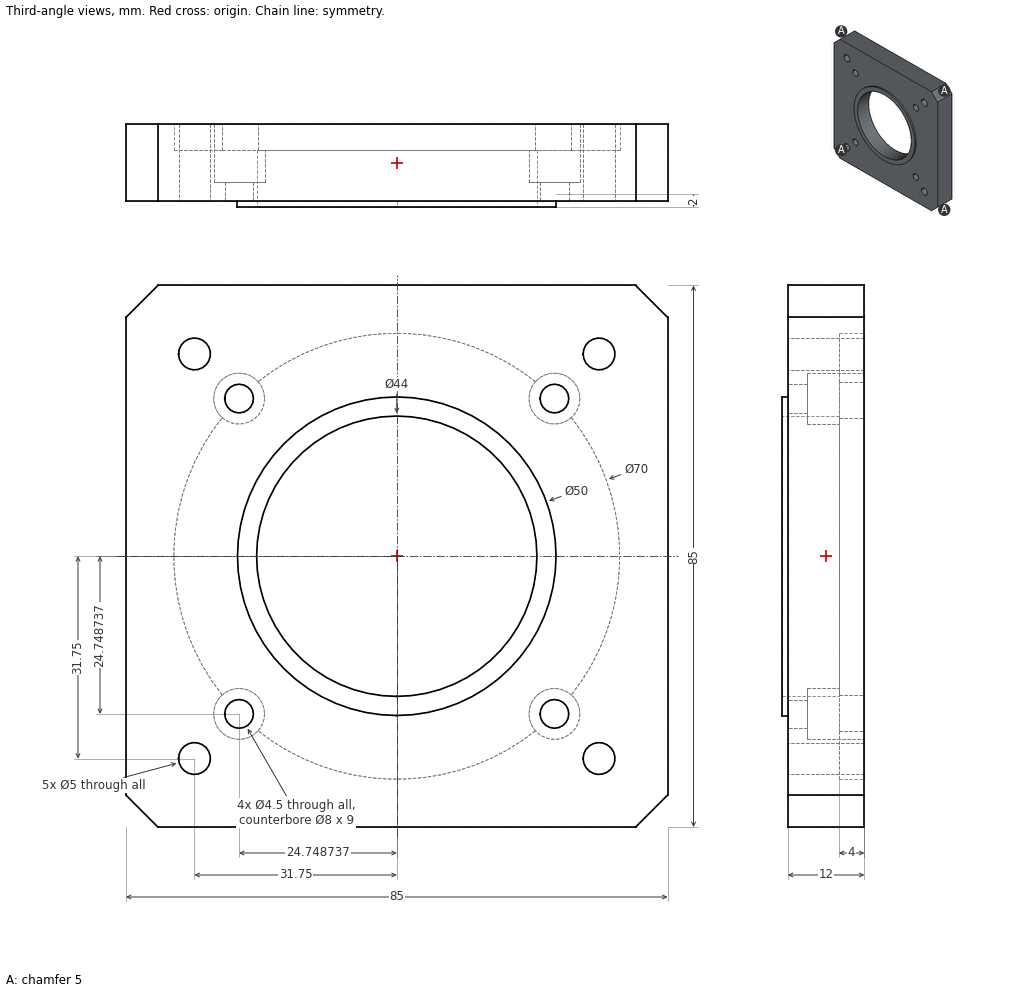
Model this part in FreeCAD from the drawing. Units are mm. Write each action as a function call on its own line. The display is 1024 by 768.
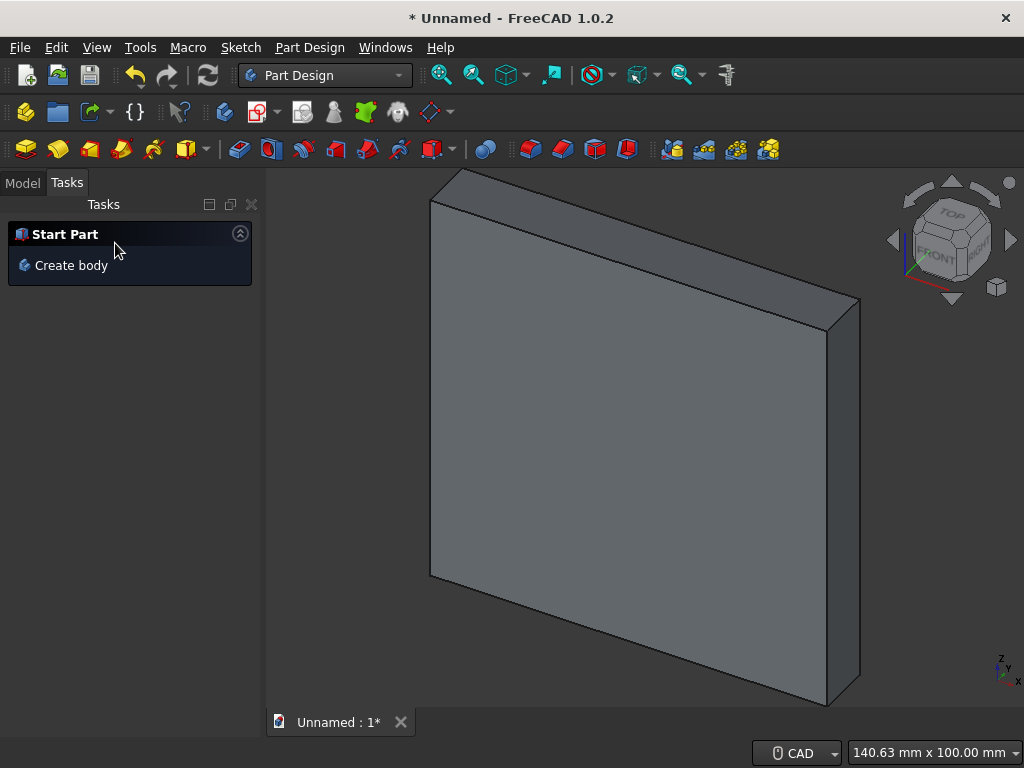
key(v)
key(f)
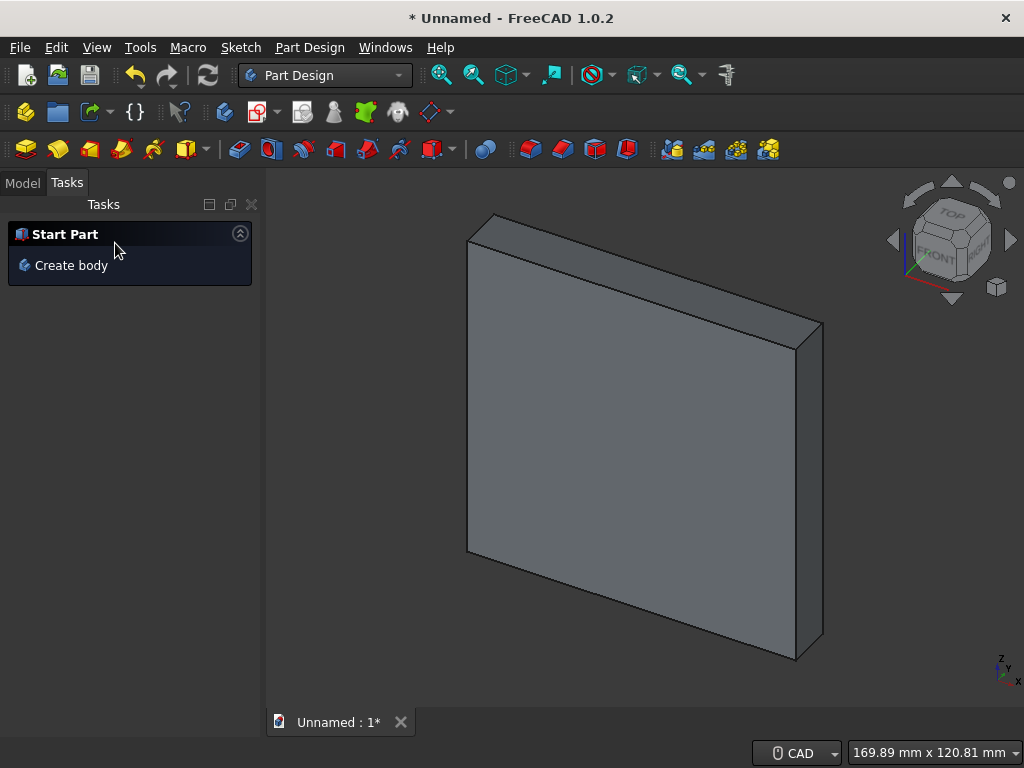
click(632, 450)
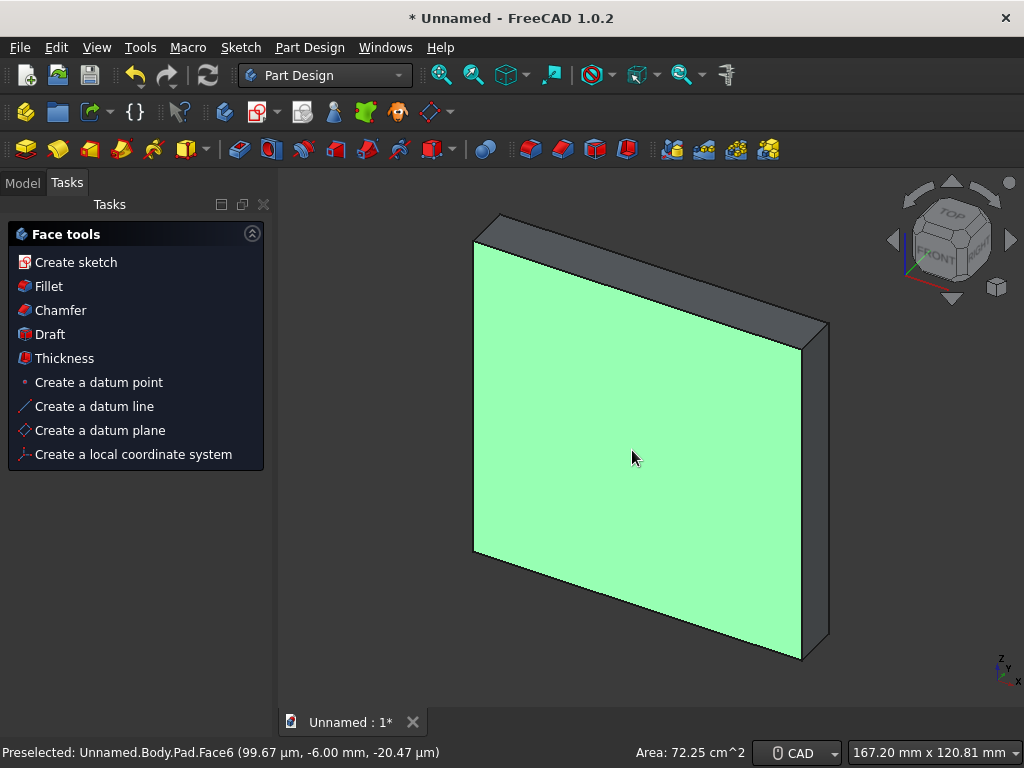
click(258, 112)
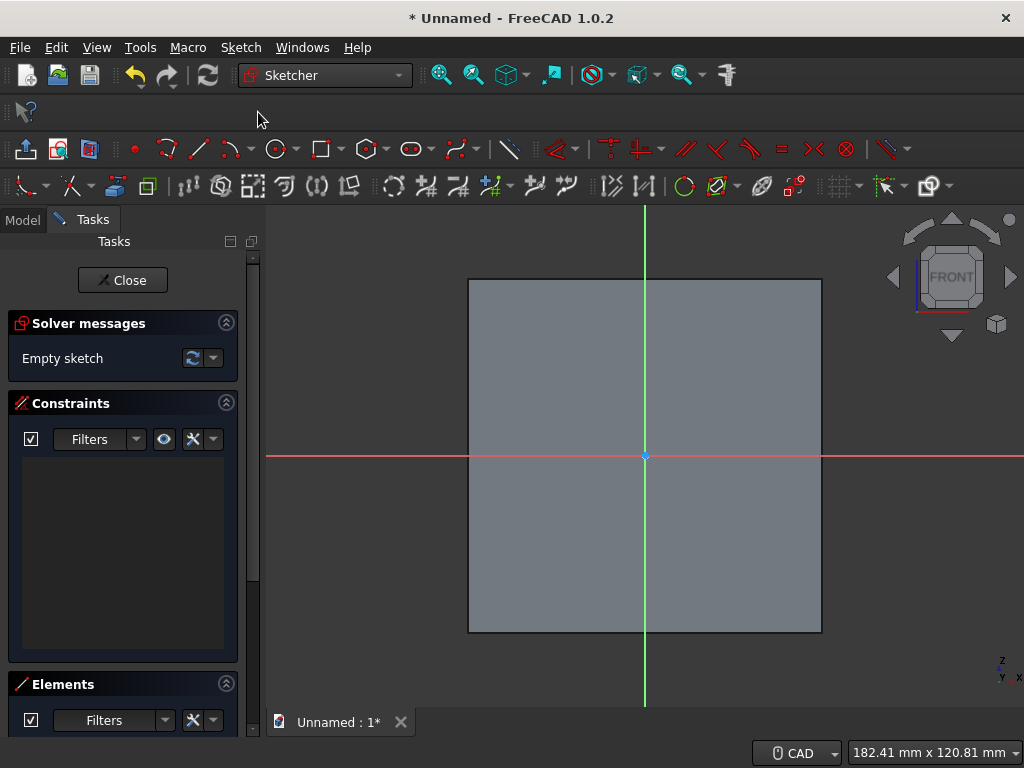
scroll(784, 456, up, 2)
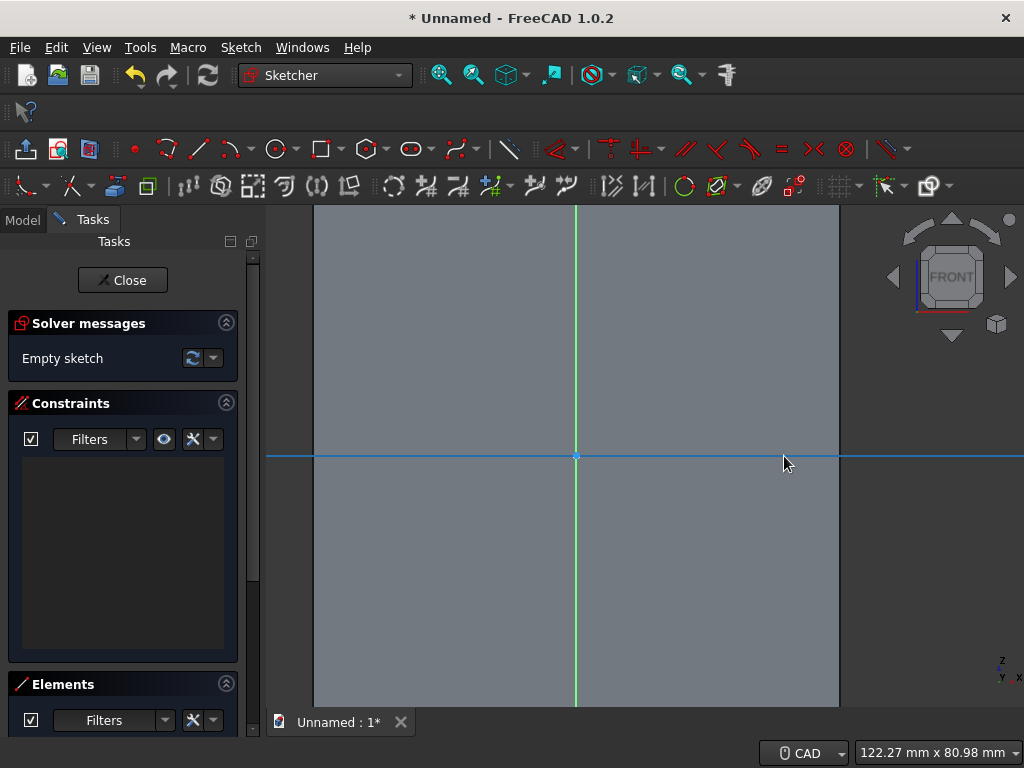
key(g)
key(c)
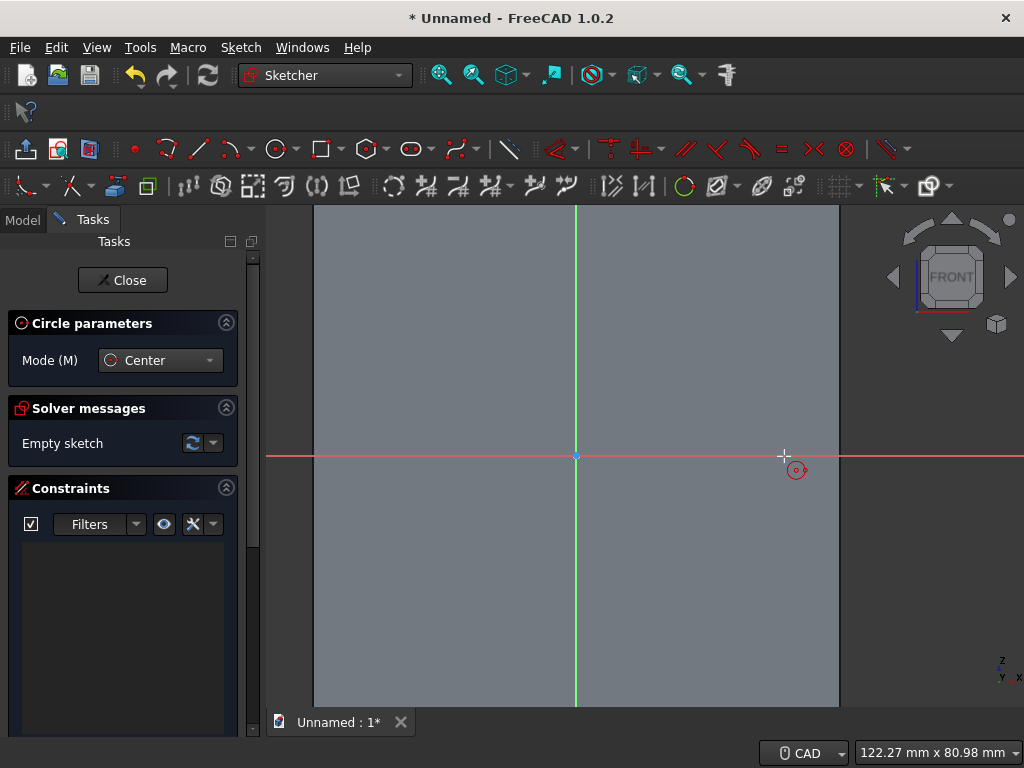
click(576, 456)
move(686, 346)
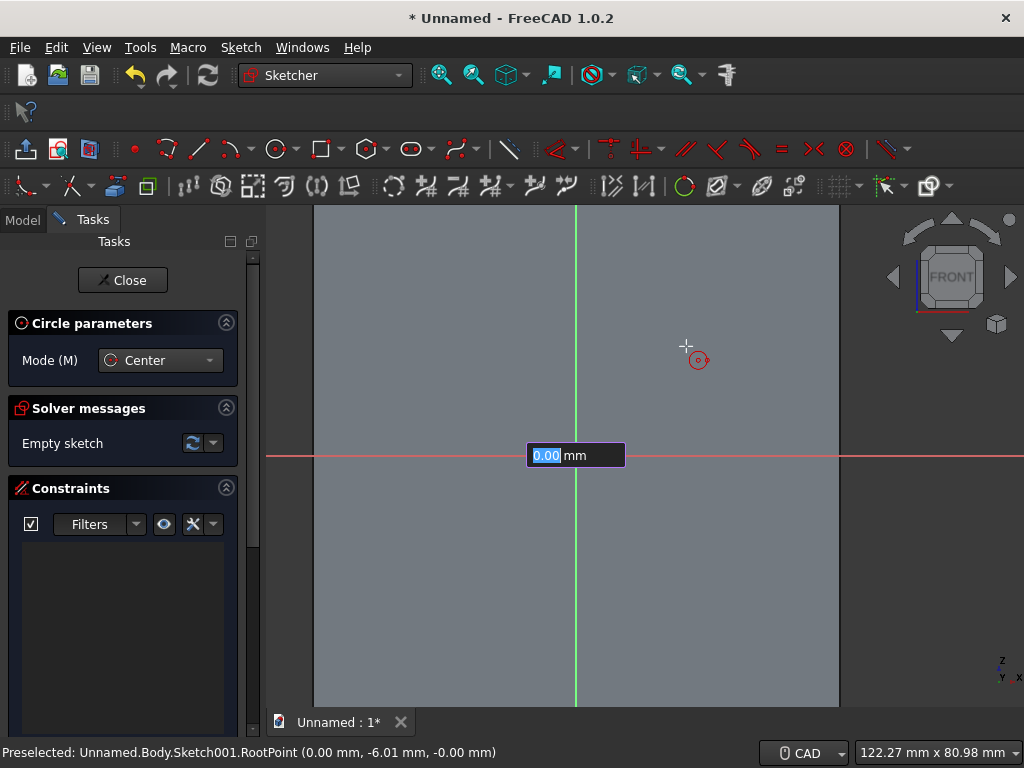
text(50)
key(Return)
key(Escape)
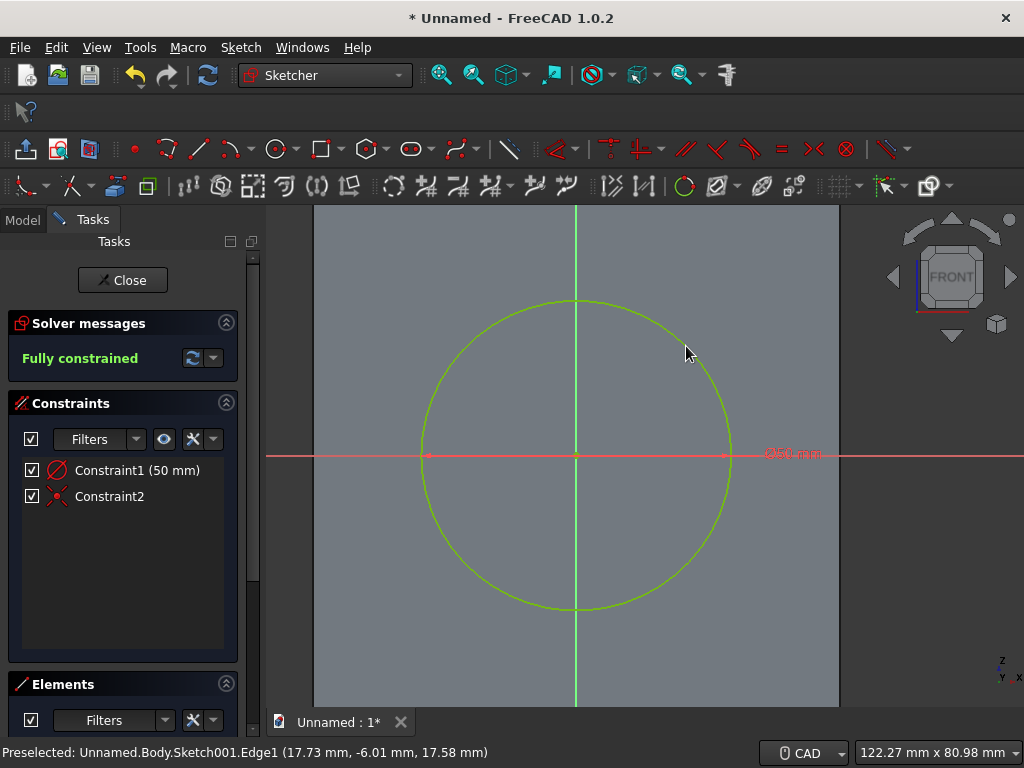
click(123, 280)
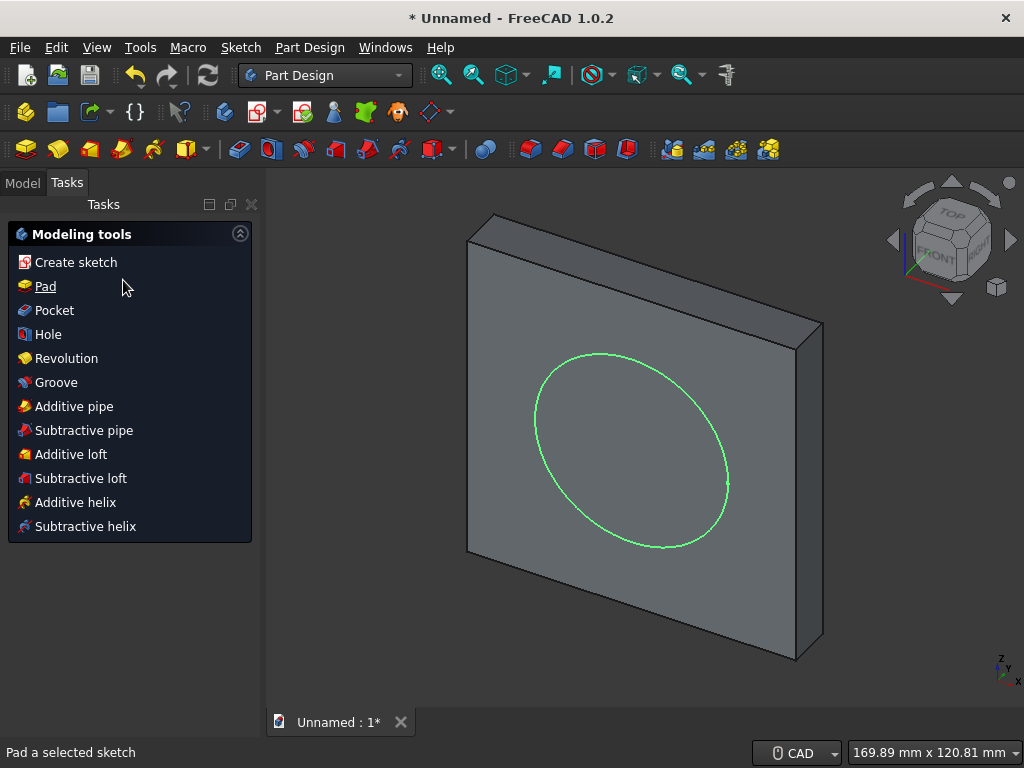
click(26, 150)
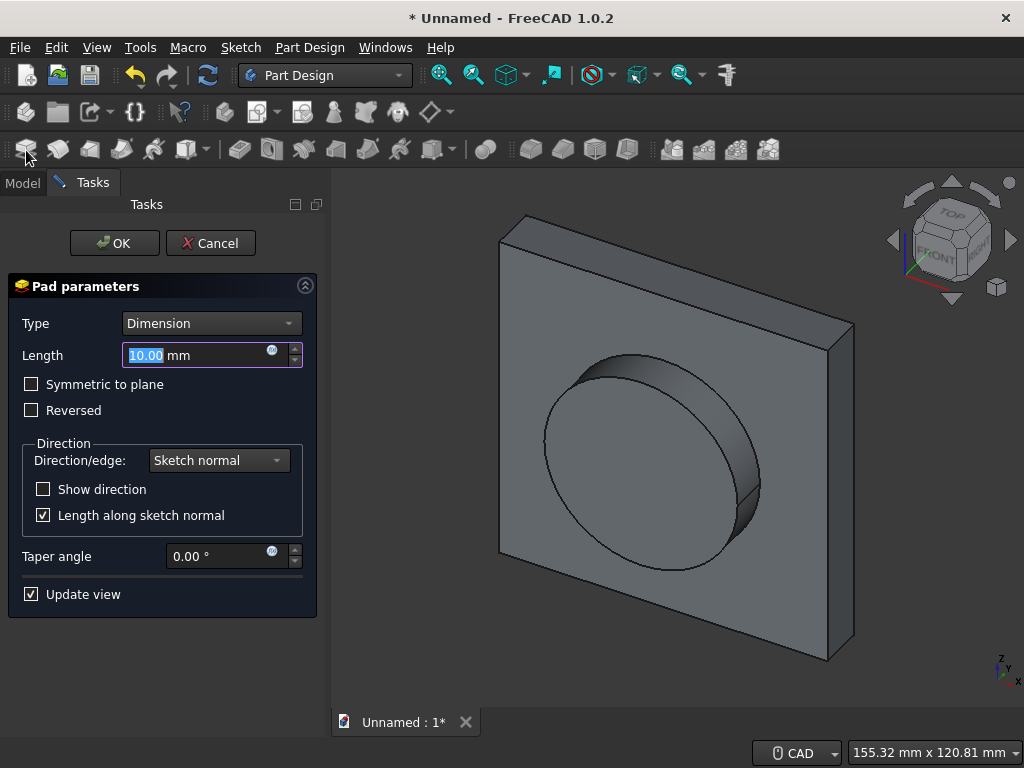
text(2)
key(Tab)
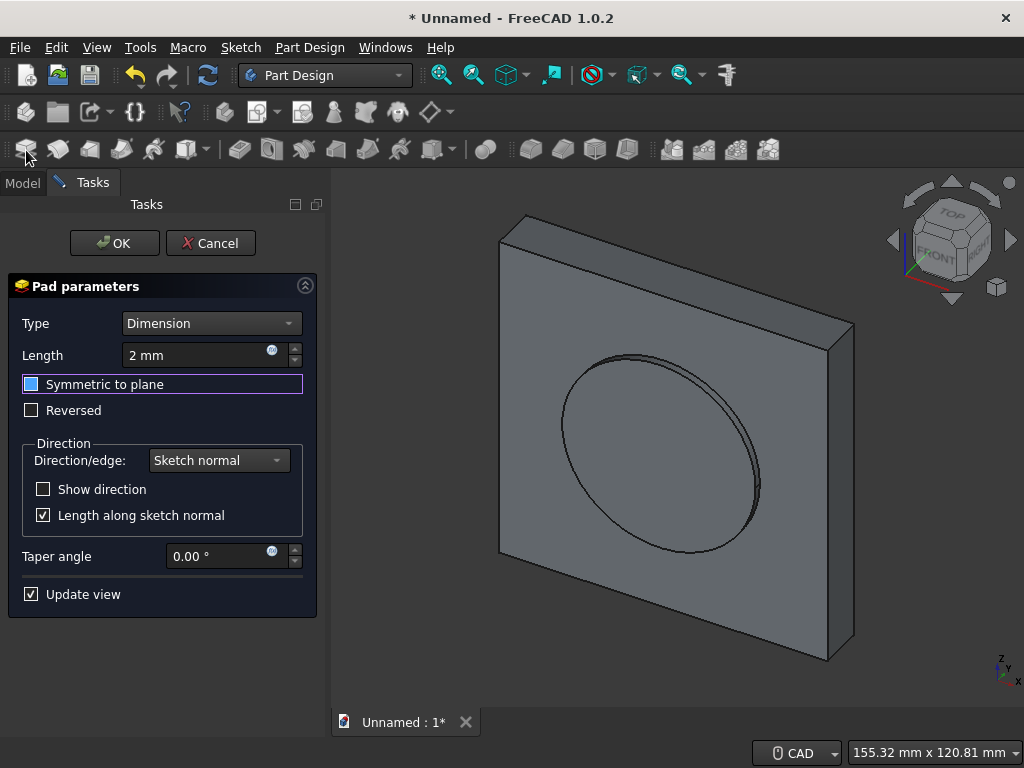
click(30, 384)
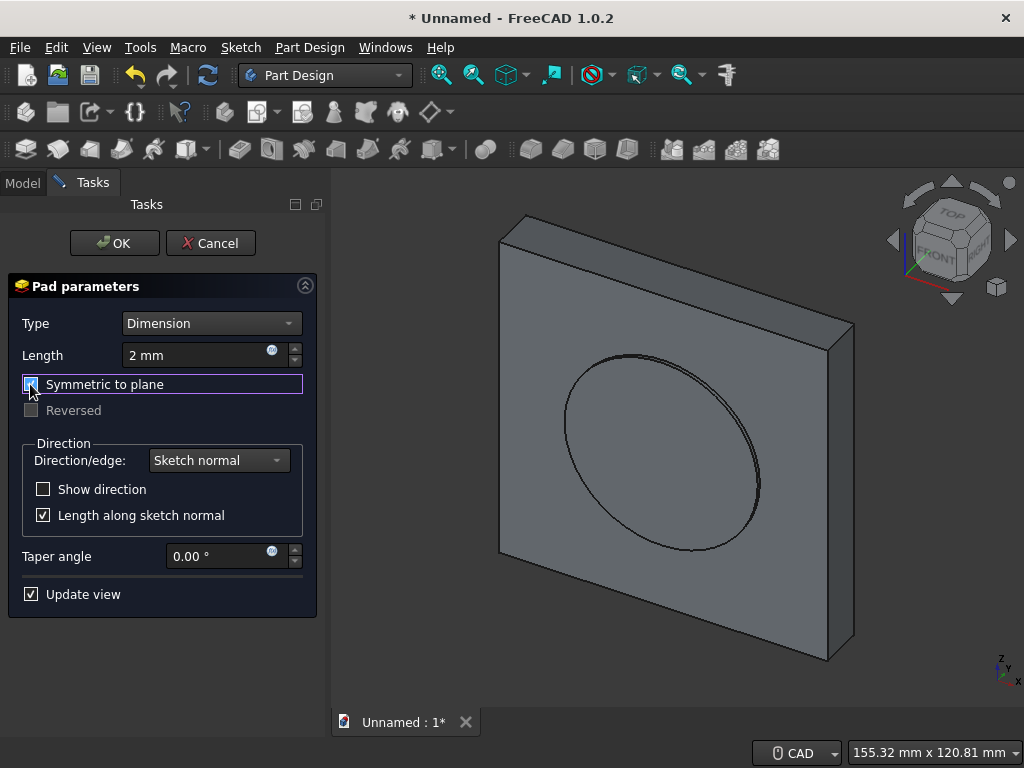
click(115, 243)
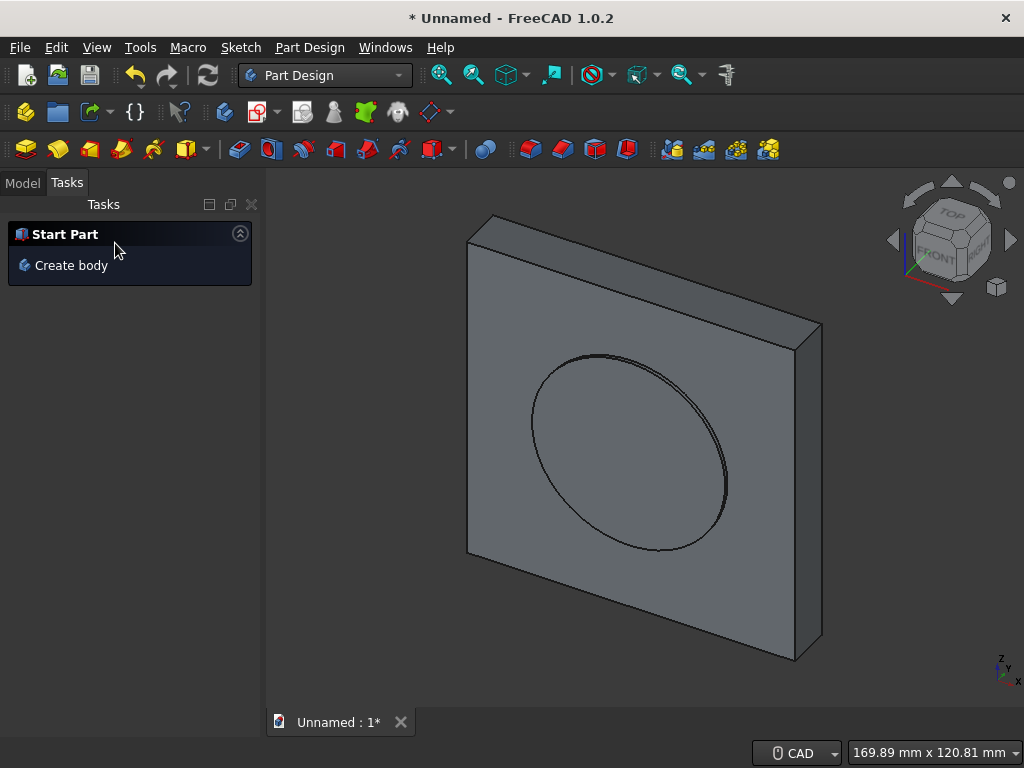
click(629, 453)